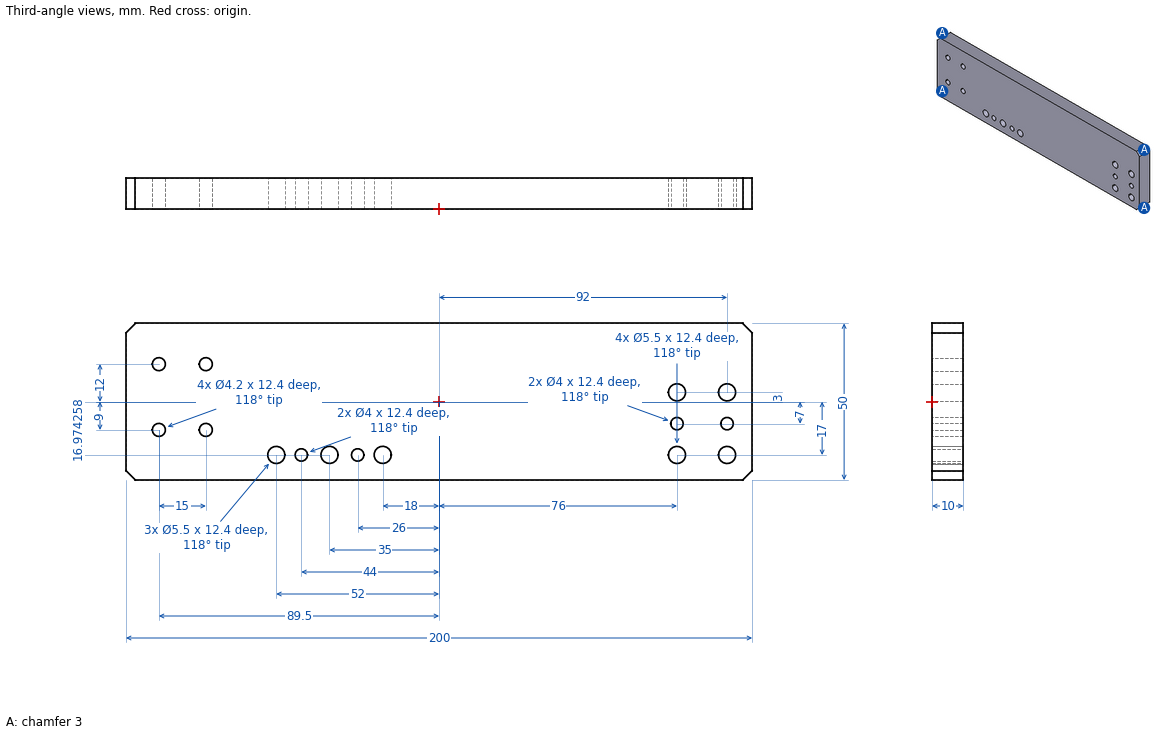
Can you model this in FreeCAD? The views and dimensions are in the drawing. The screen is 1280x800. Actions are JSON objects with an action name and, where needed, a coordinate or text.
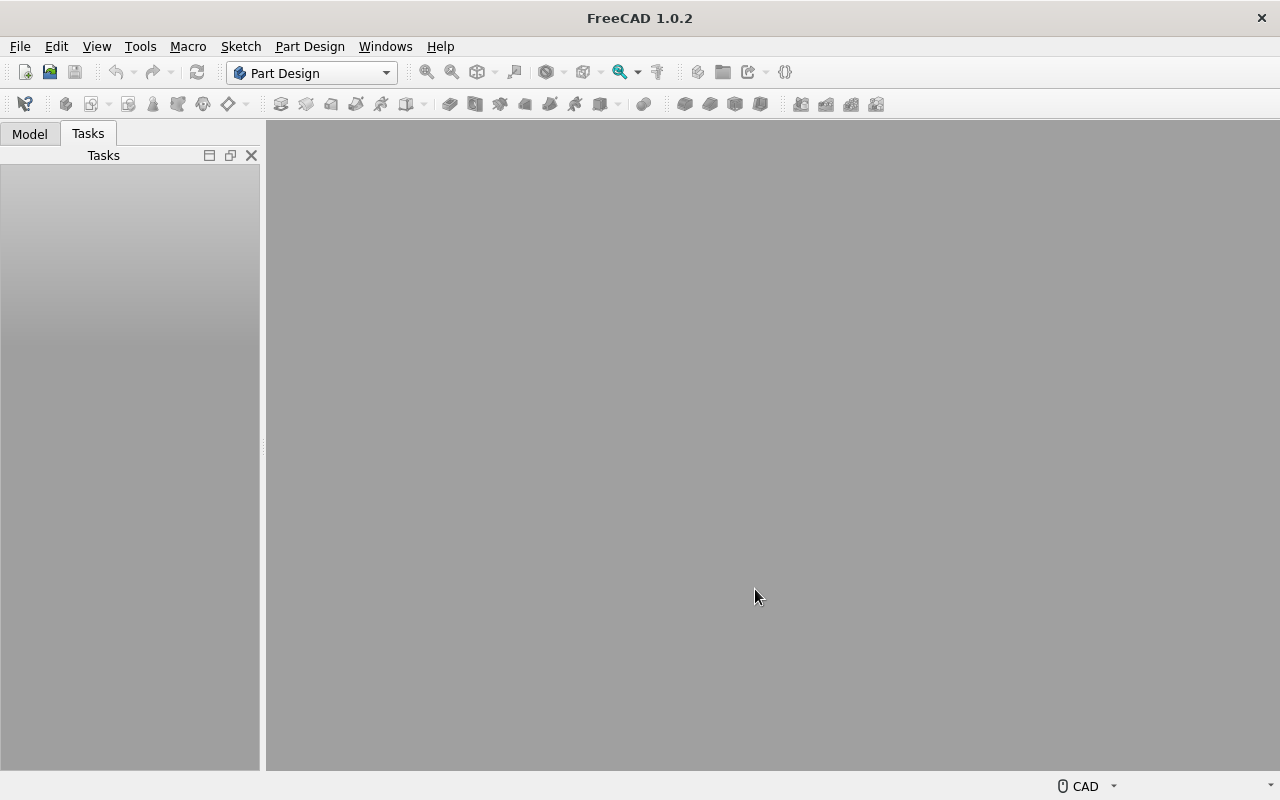
{"action": "key", "text": "ctrl+n"}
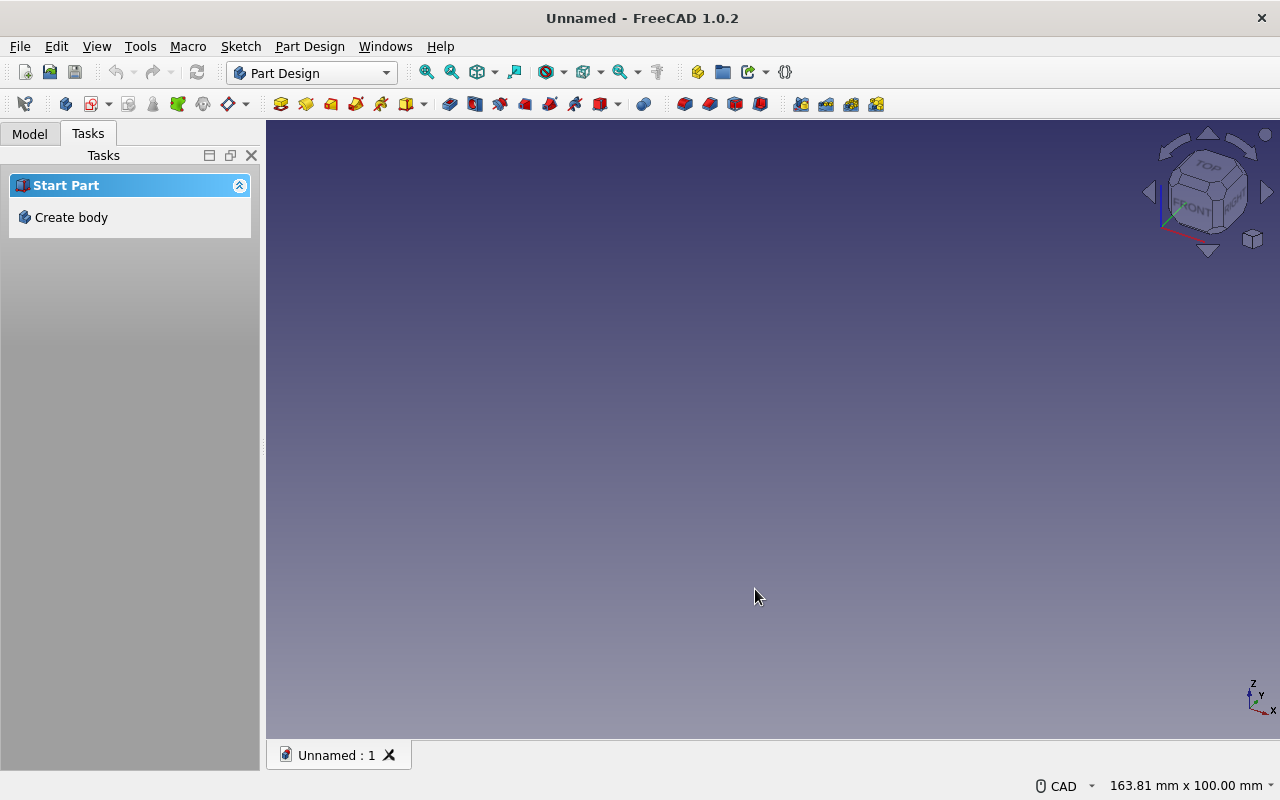
{"action": "left_click", "coordinate": [90, 104]}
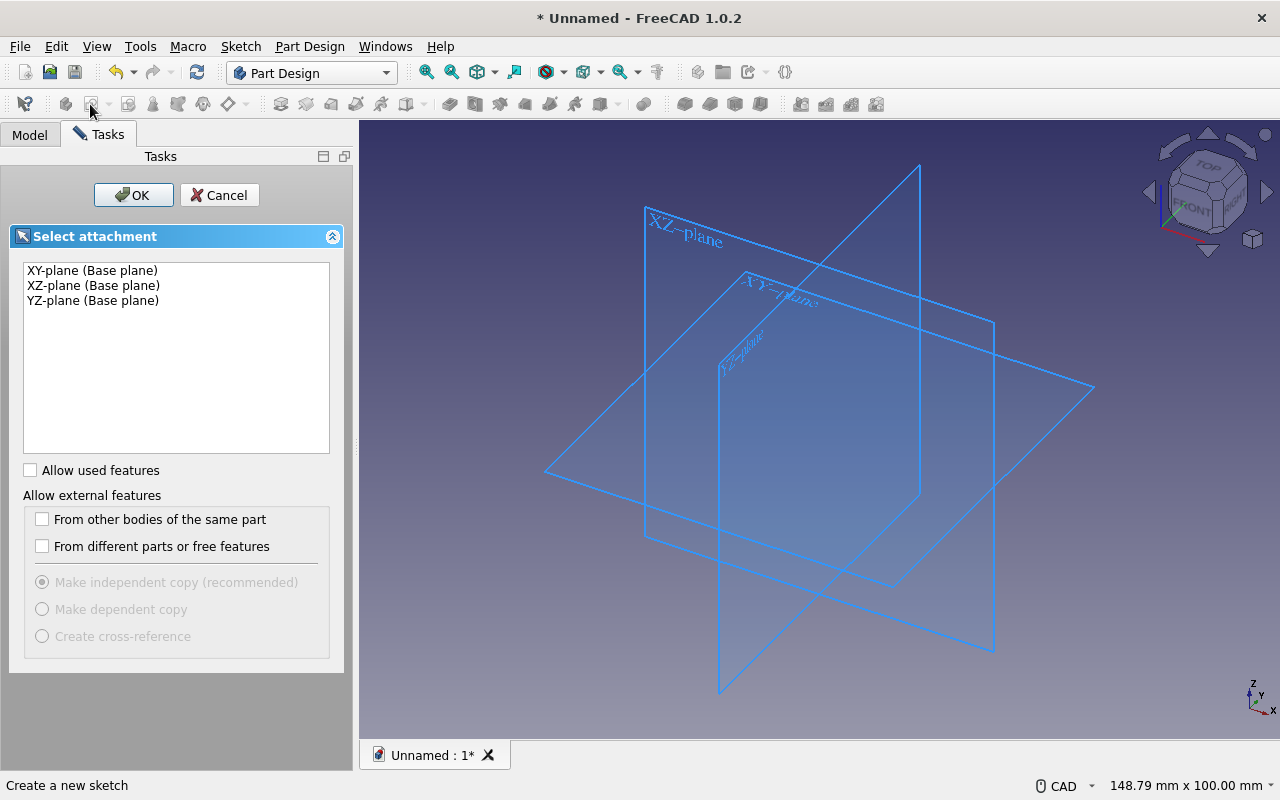
{"action": "left_click", "coordinate": [84, 286]}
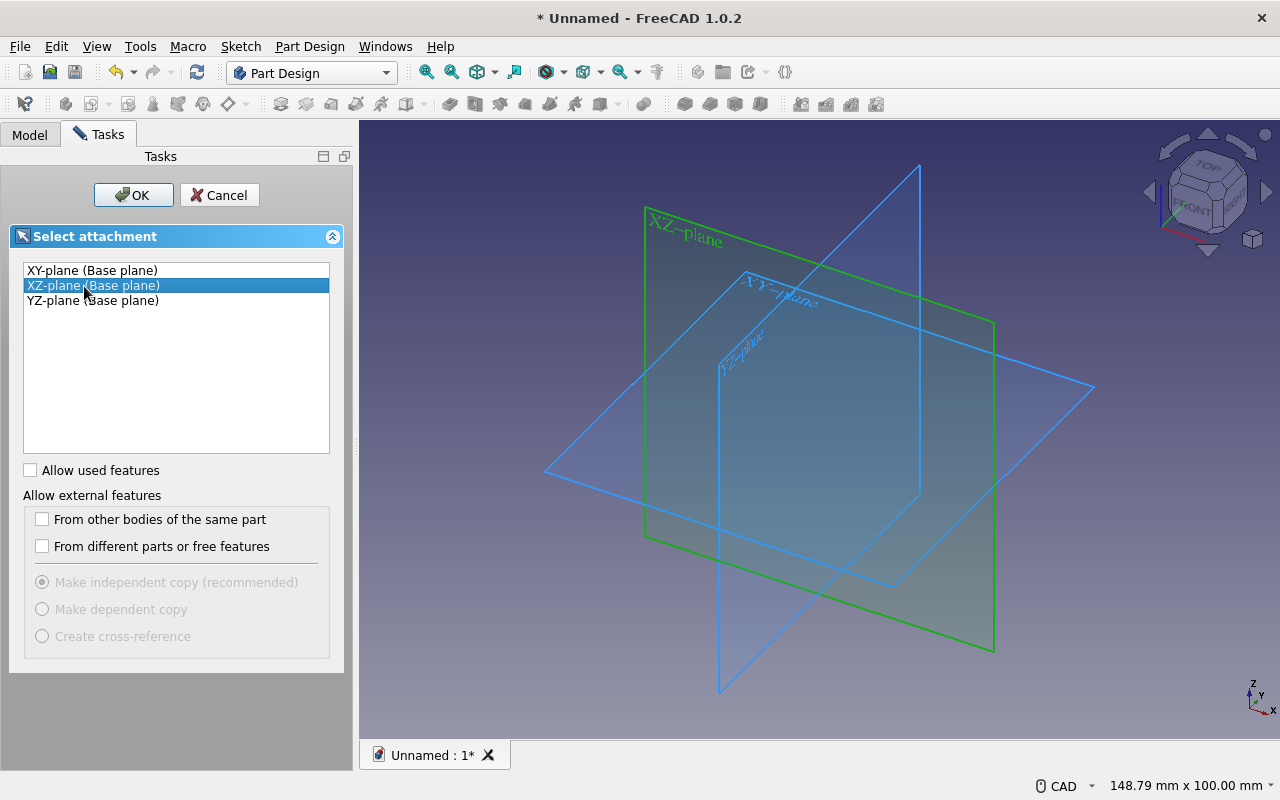
{"action": "left_click", "coordinate": [134, 195]}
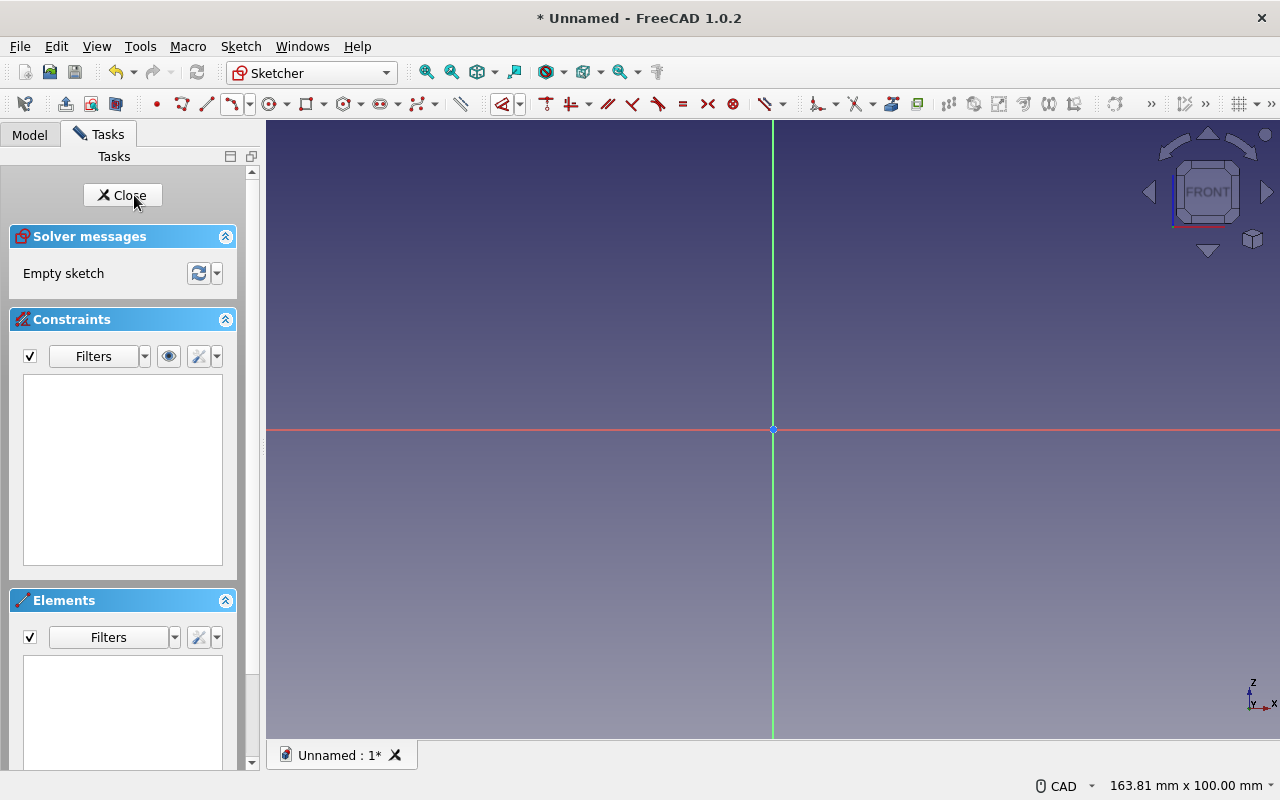
{"action": "scroll", "coordinate": [649, 430], "scroll_direction": "down", "scroll_amount": 4}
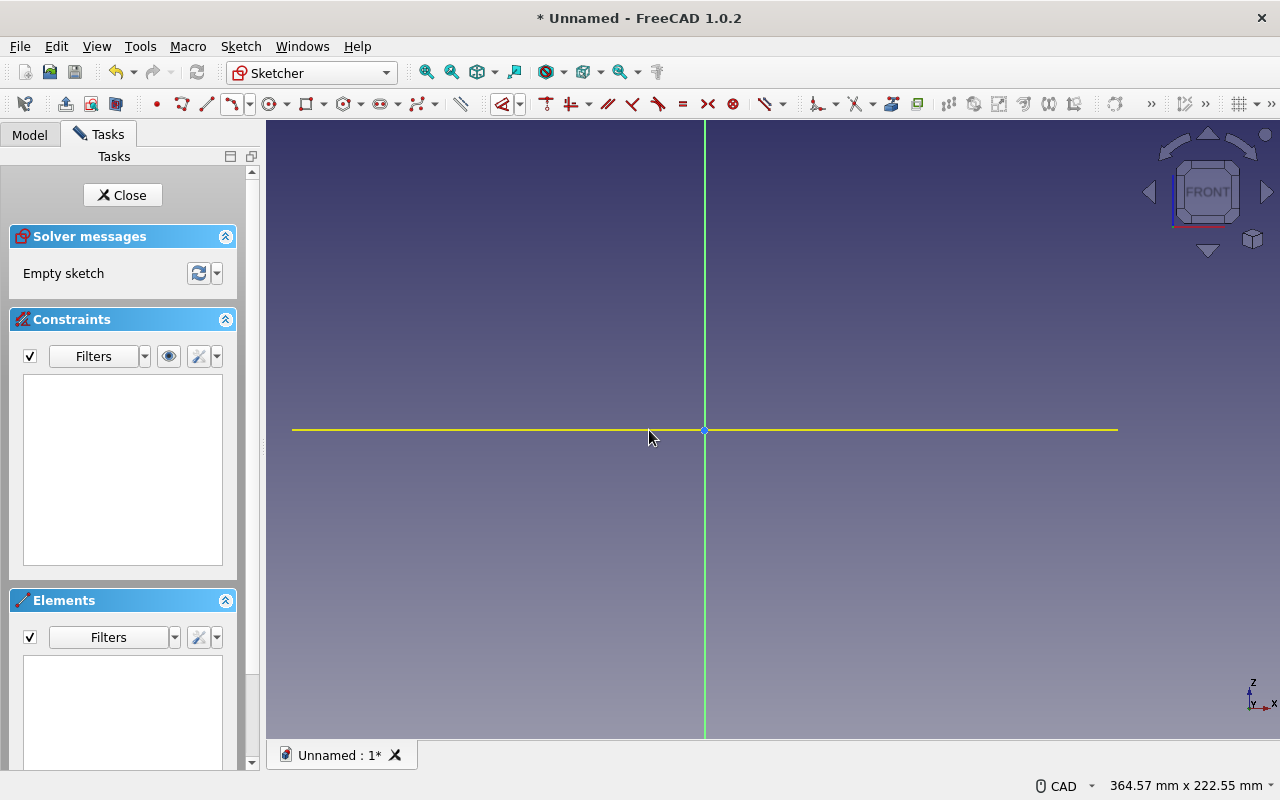
{"action": "key", "text": "g v"}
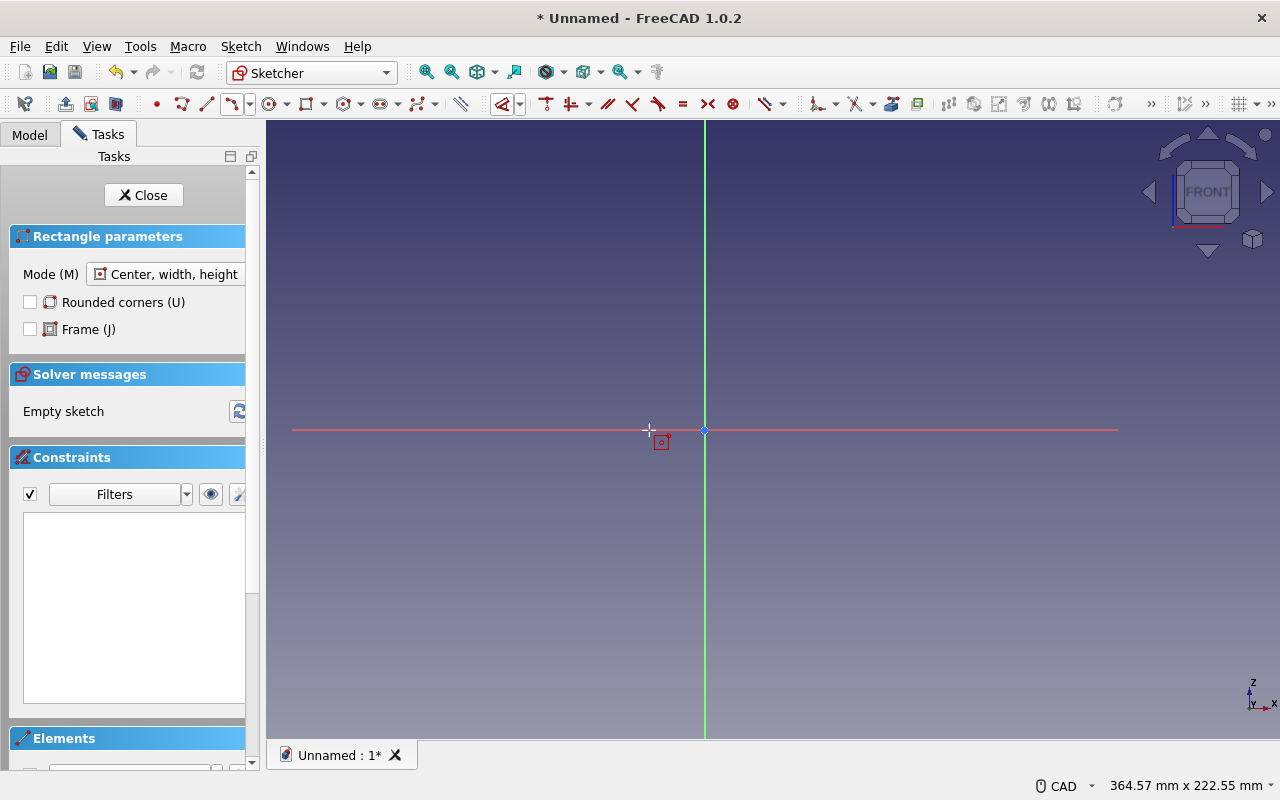
{"action": "left_click", "coordinate": [705, 430]}
{"action": "left_click", "coordinate": [983, 361]}
{"action": "key", "text": "Escape"}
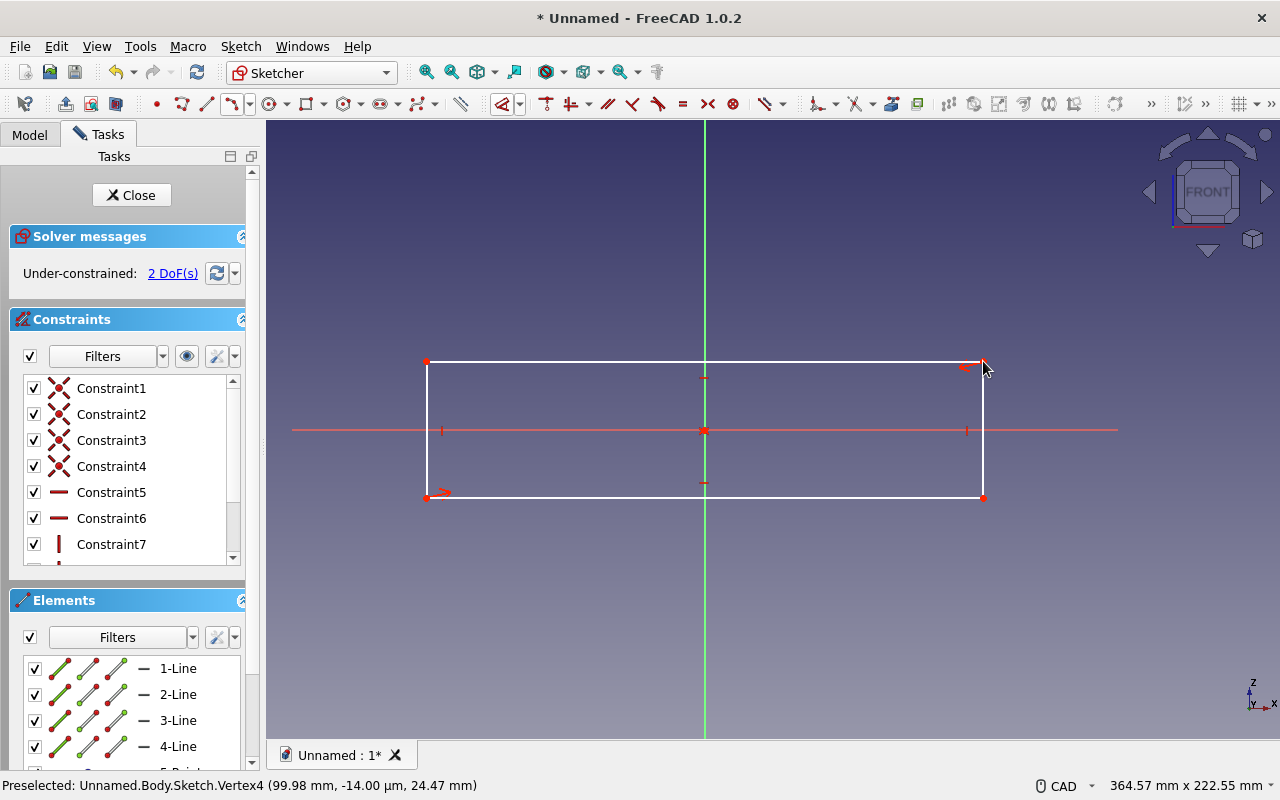
{"action": "key", "text": "d"}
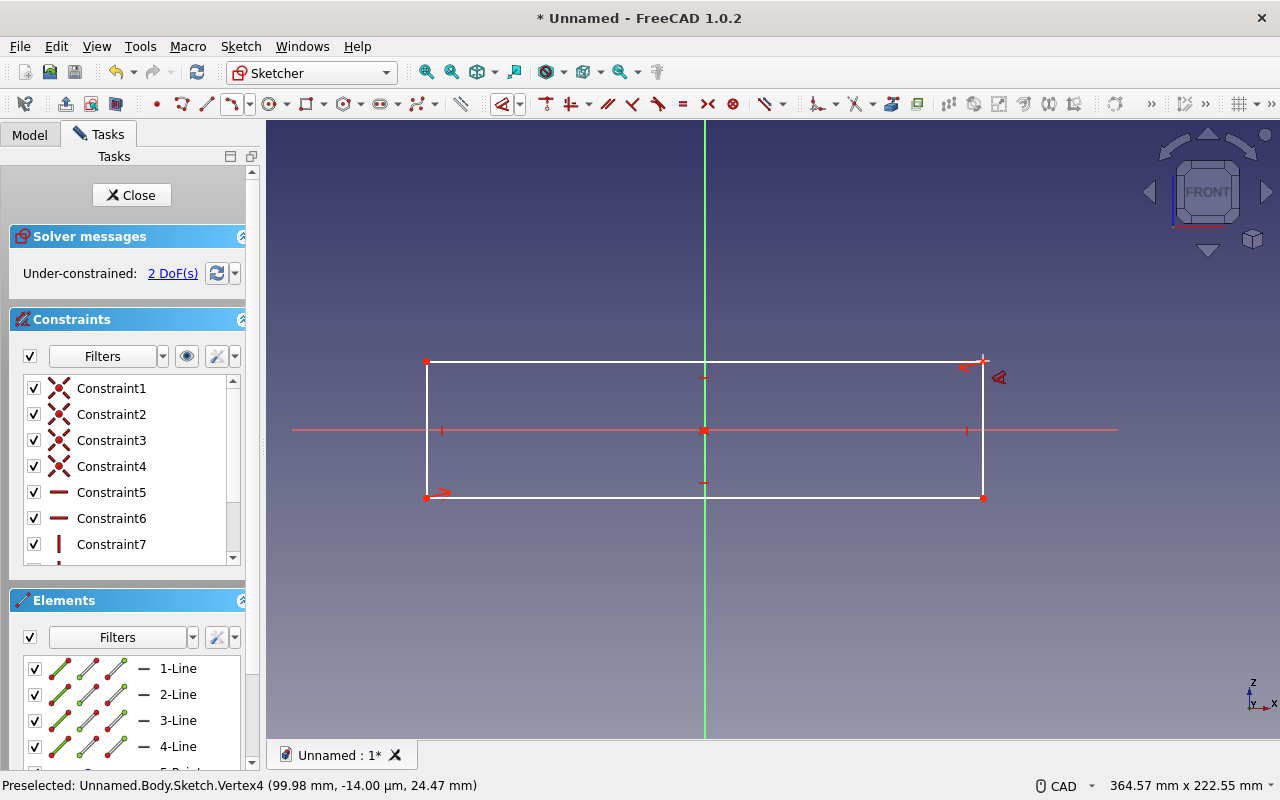
{"action": "left_click", "coordinate": [983, 457]}
{"action": "left_click", "coordinate": [1017, 399]}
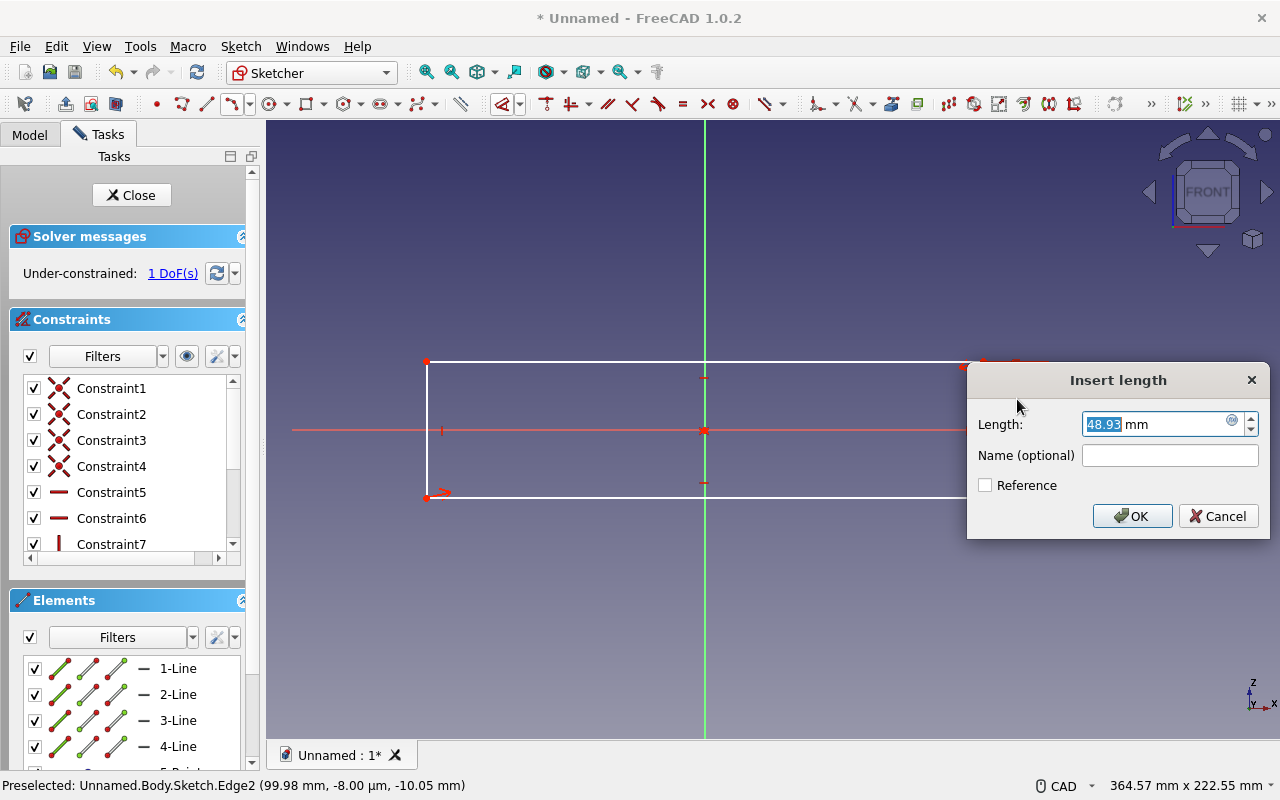
{"action": "type", "text": "50"}
{"action": "key", "text": "Return"}